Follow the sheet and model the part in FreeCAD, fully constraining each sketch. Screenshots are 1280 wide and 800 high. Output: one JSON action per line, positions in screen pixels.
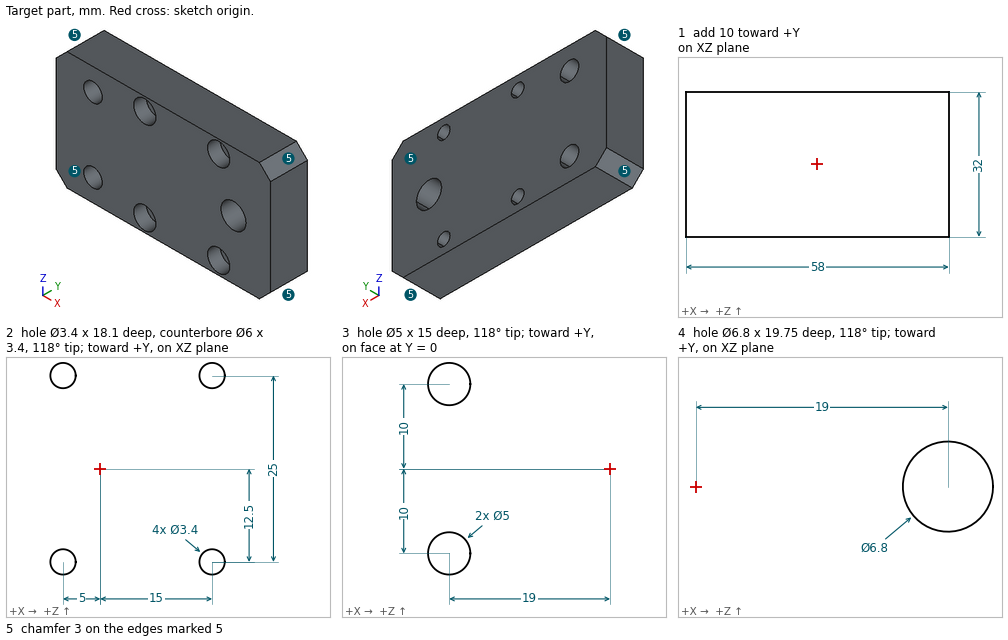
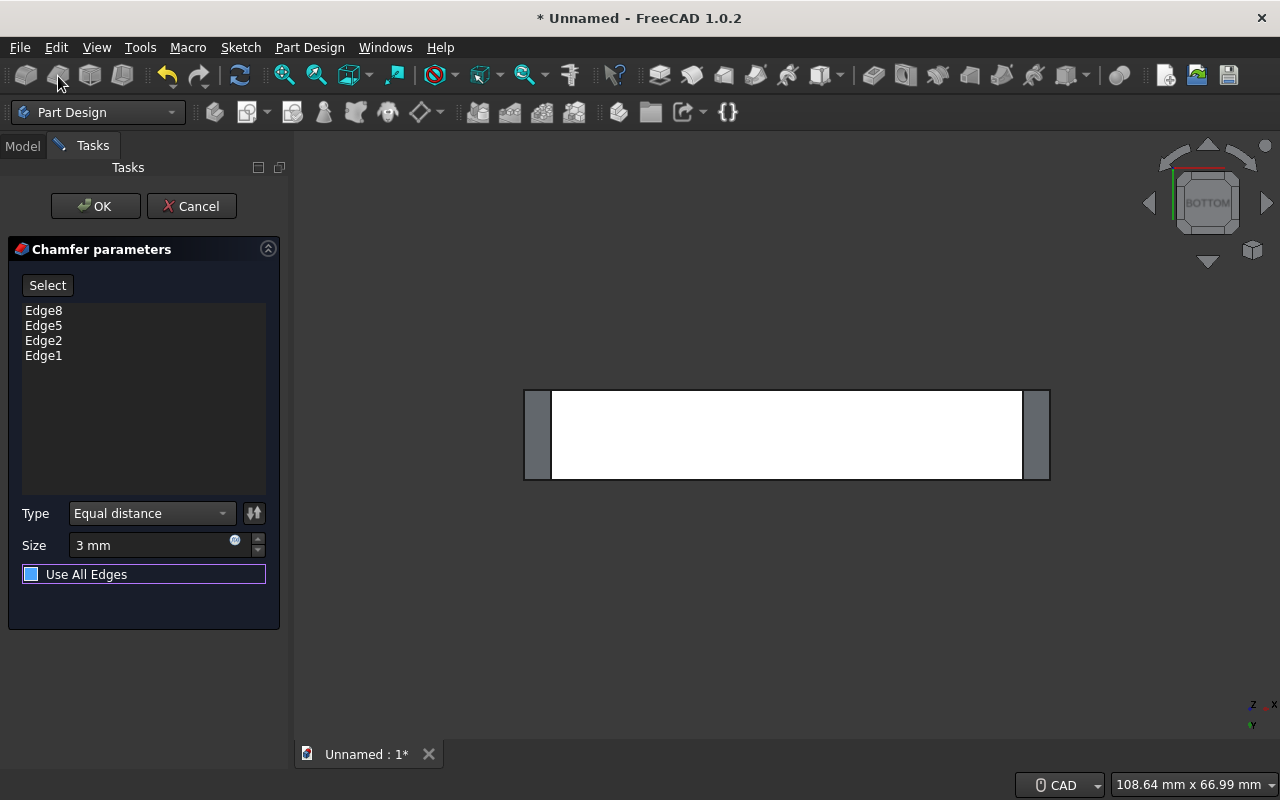
{"action": "left_click", "coordinate": [96, 206]}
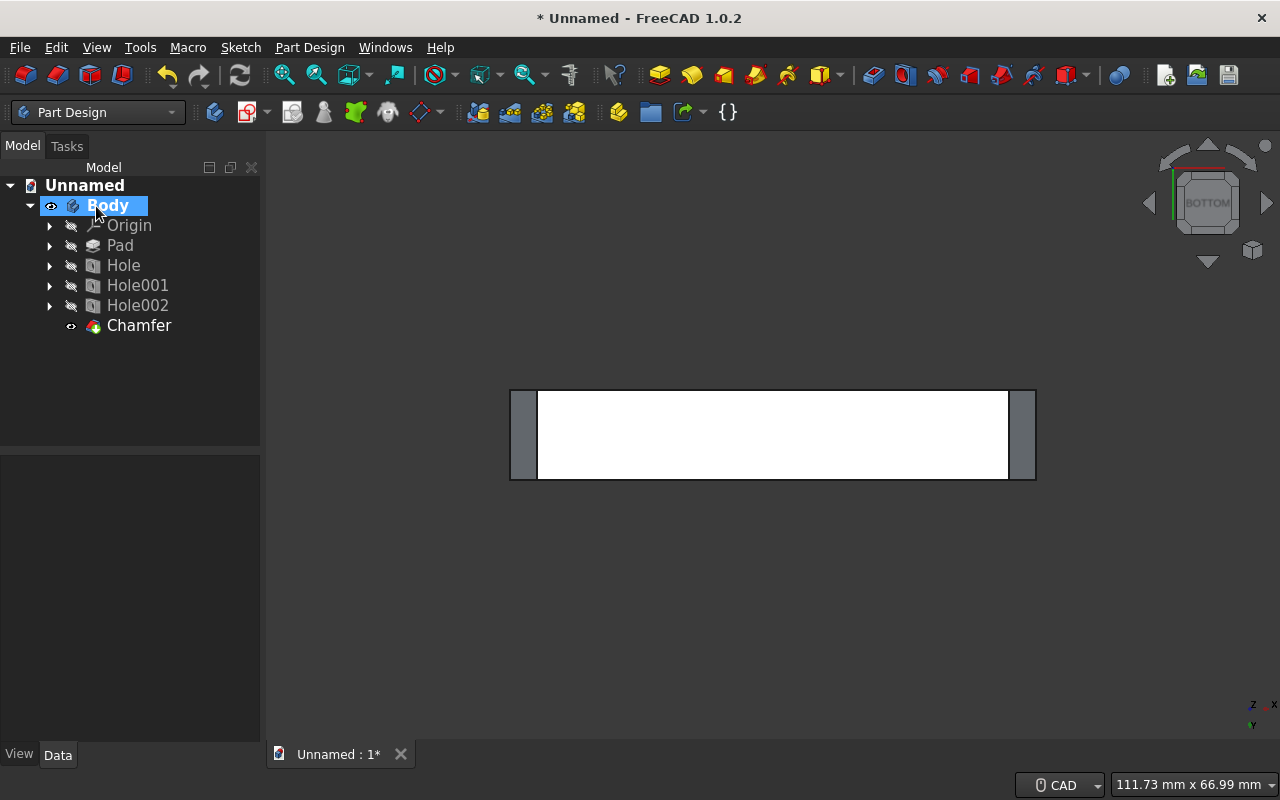
{"action": "key", "text": "0"}